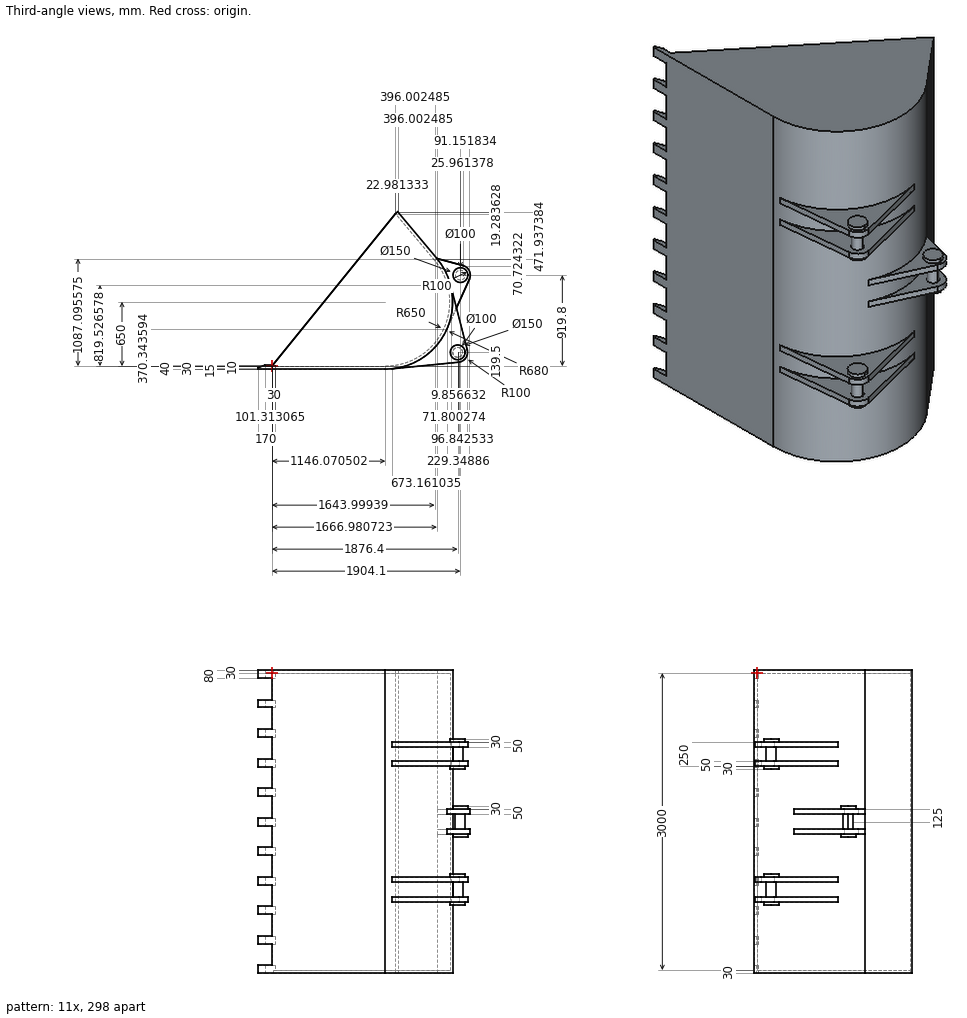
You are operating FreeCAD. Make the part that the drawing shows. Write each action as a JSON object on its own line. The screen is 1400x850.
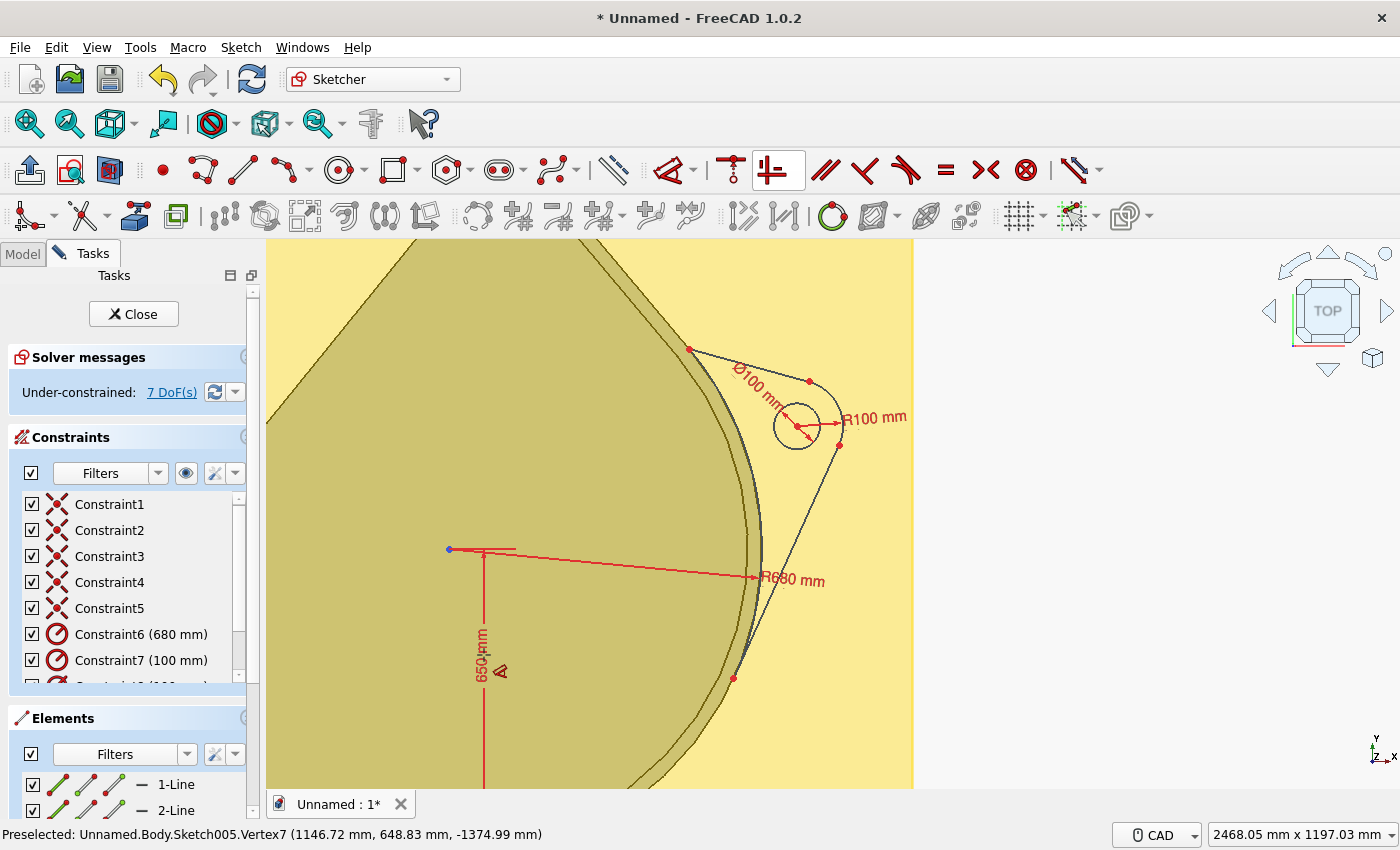
{"action": "left_click", "coordinate": [797, 426]}
{"action": "left_click", "coordinate": [831, 517]}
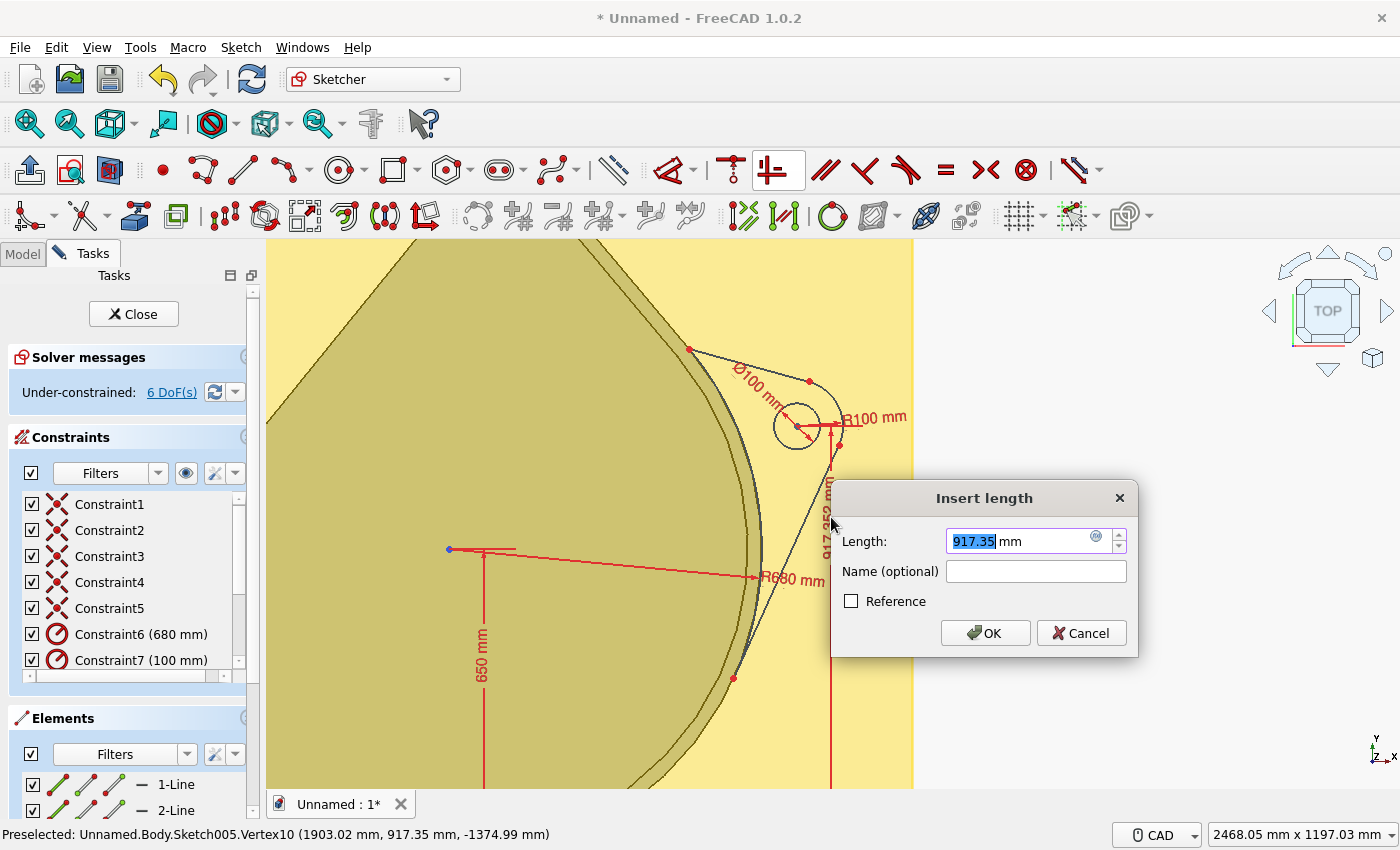
{"action": "type", "text": "919.8"}
{"action": "key", "text": "Return"}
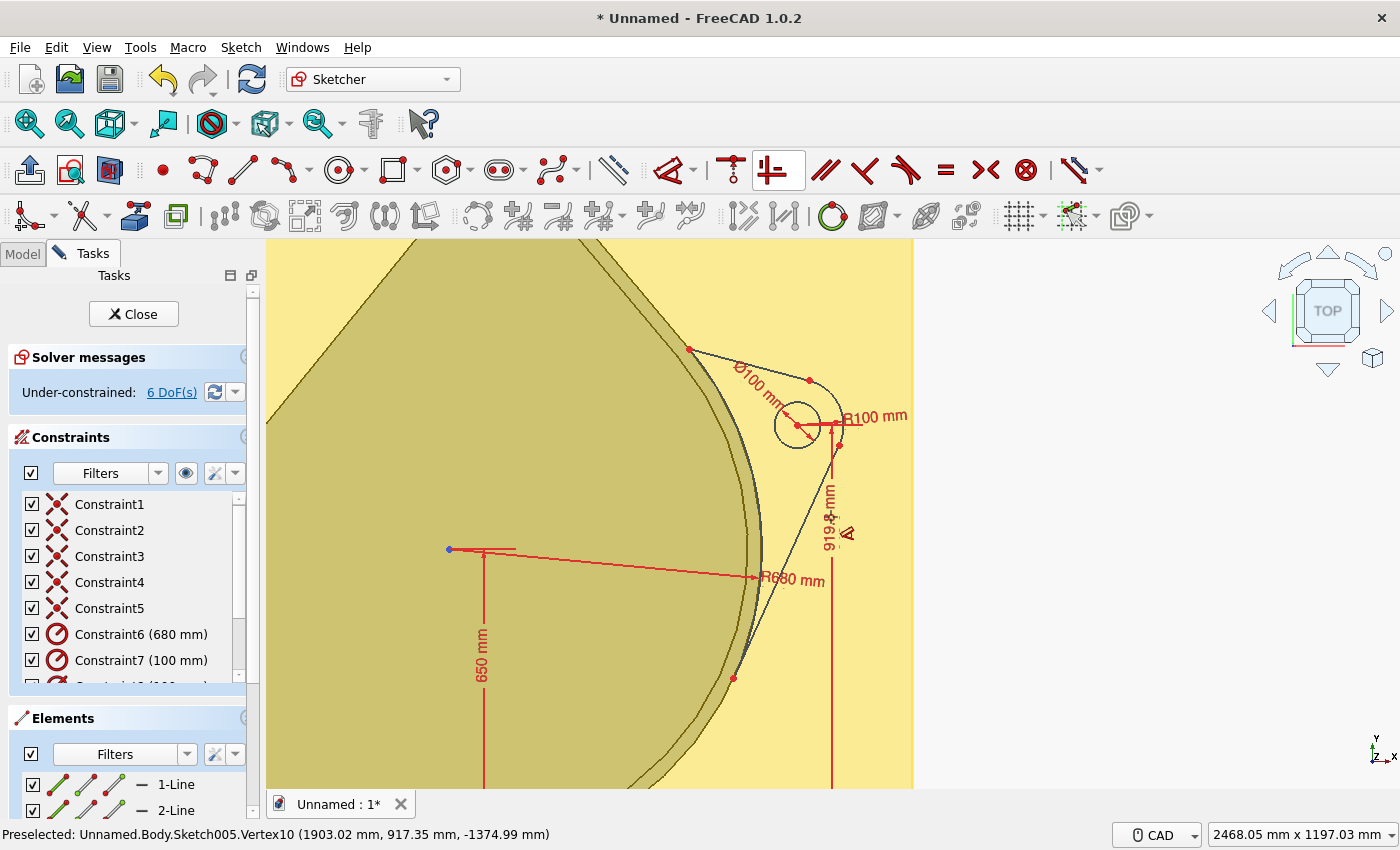
{"action": "left_click", "coordinate": [798, 425]}
{"action": "left_click", "coordinate": [546, 391]}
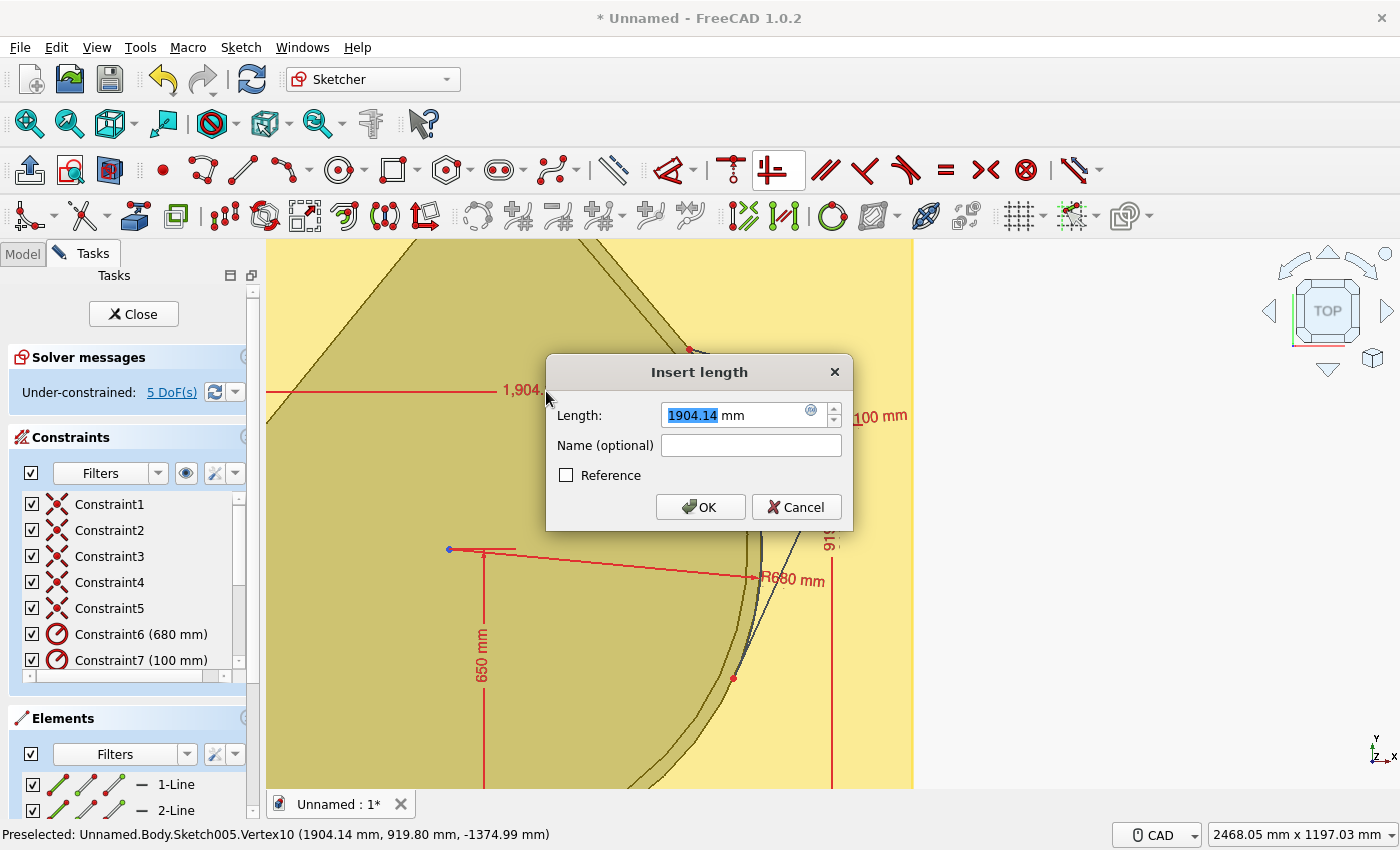
{"action": "type", "text": "1904.1"}
{"action": "key", "text": "Return"}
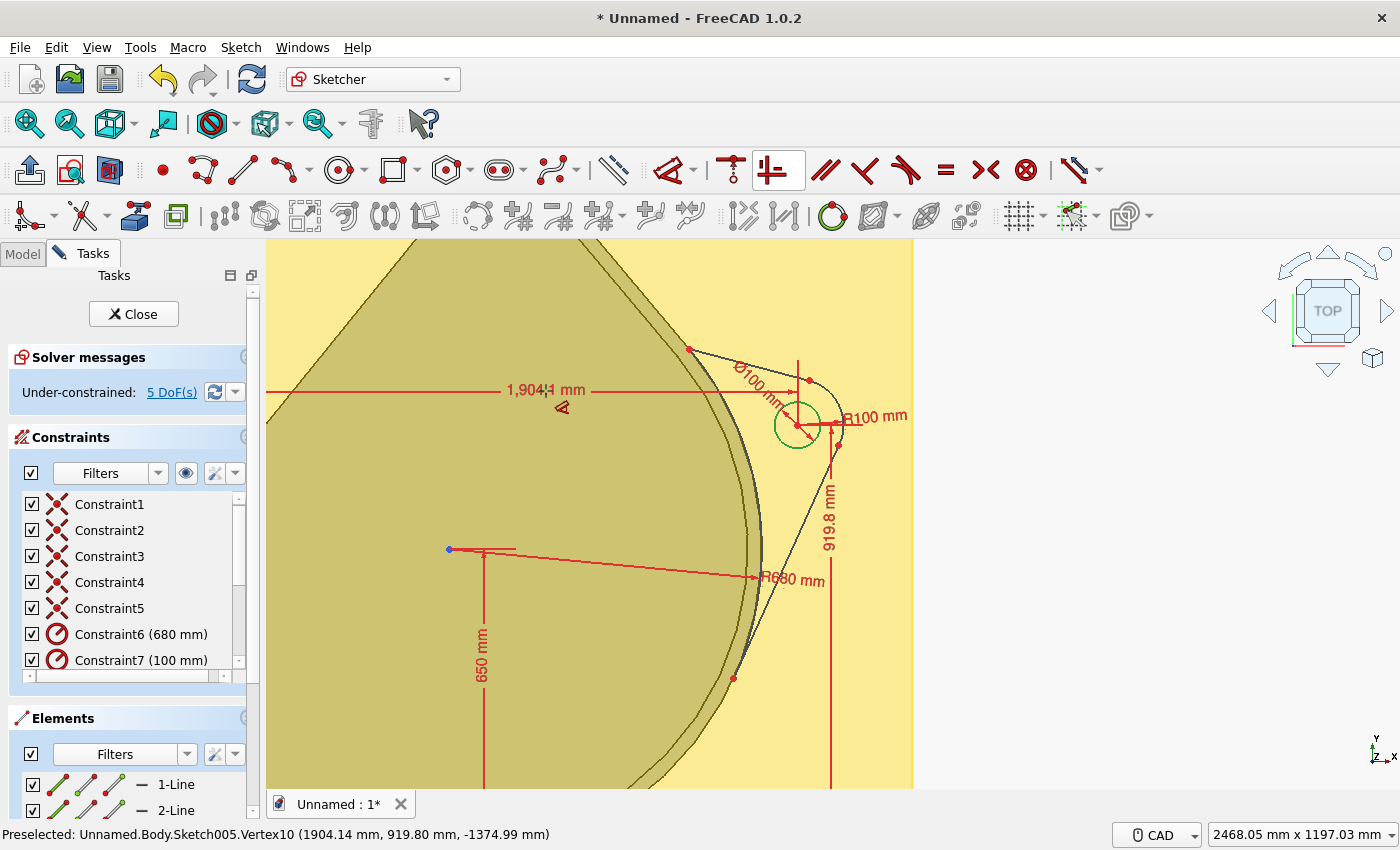
{"action": "scroll", "coordinate": [773, 371], "scroll_direction": "up", "scroll_amount": 2}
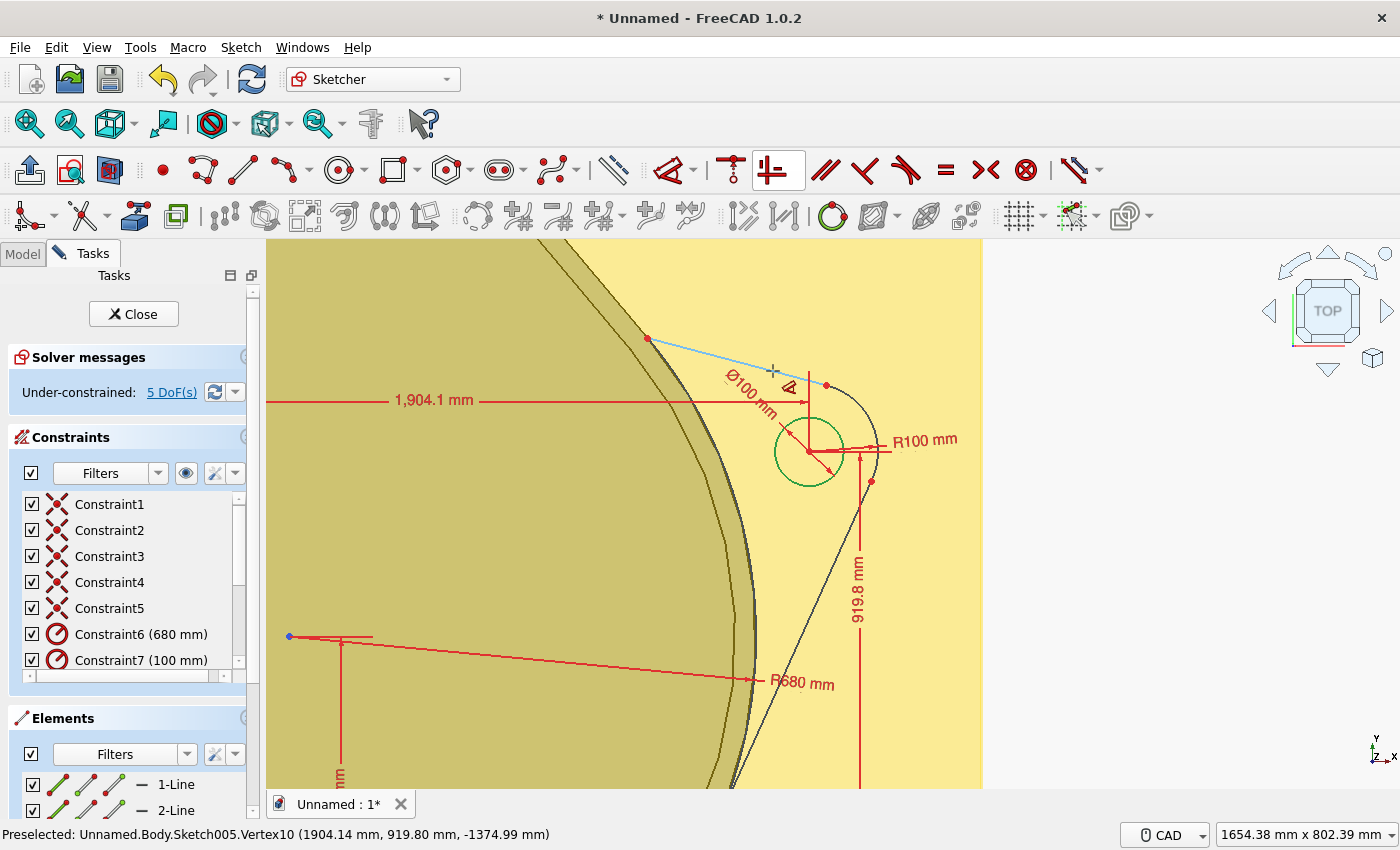
{"action": "left_click", "coordinate": [773, 371]}
{"action": "left_click", "coordinate": [614, 362]}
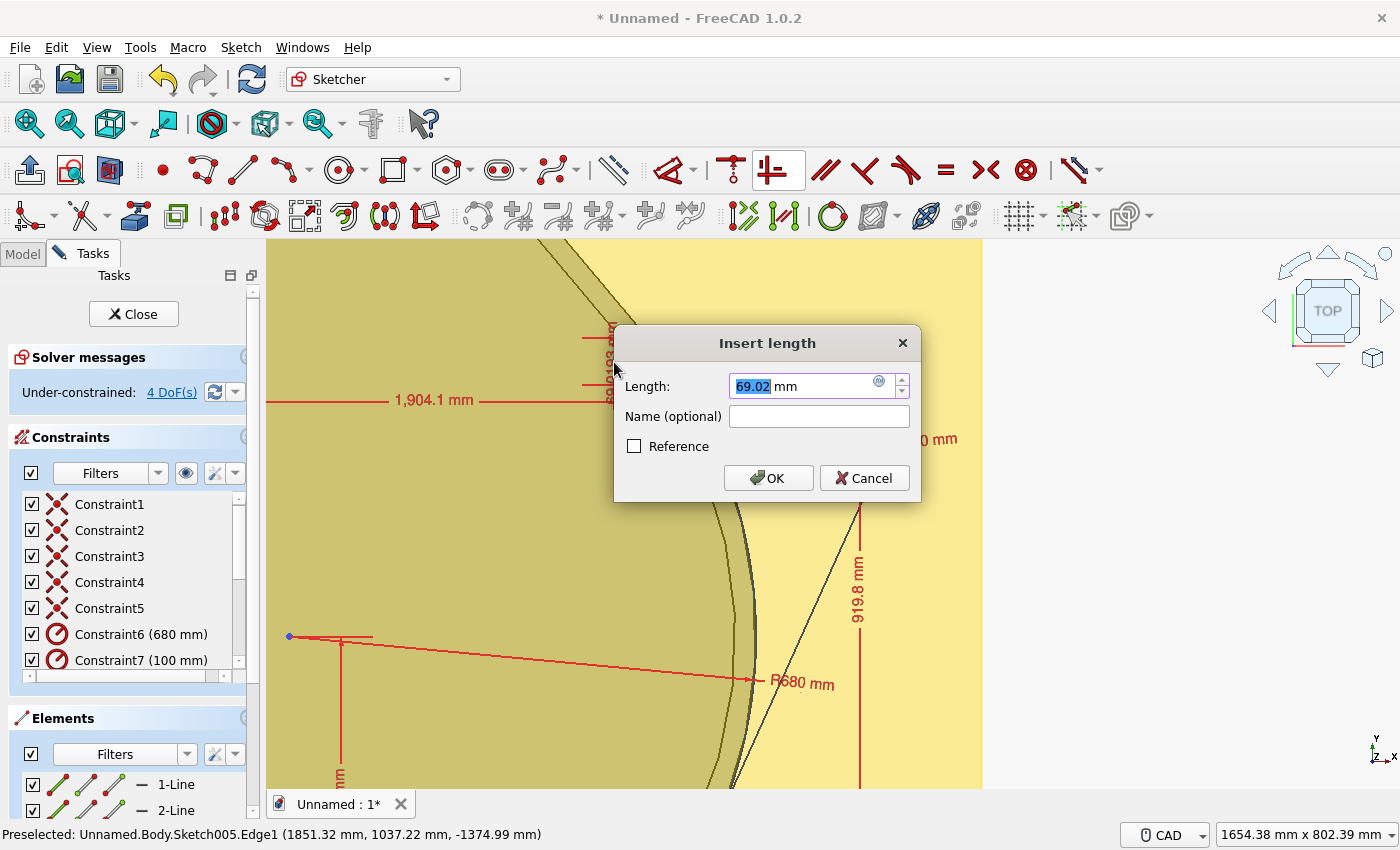
{"action": "type", "text": "70.724322"}
{"action": "key", "text": "Return"}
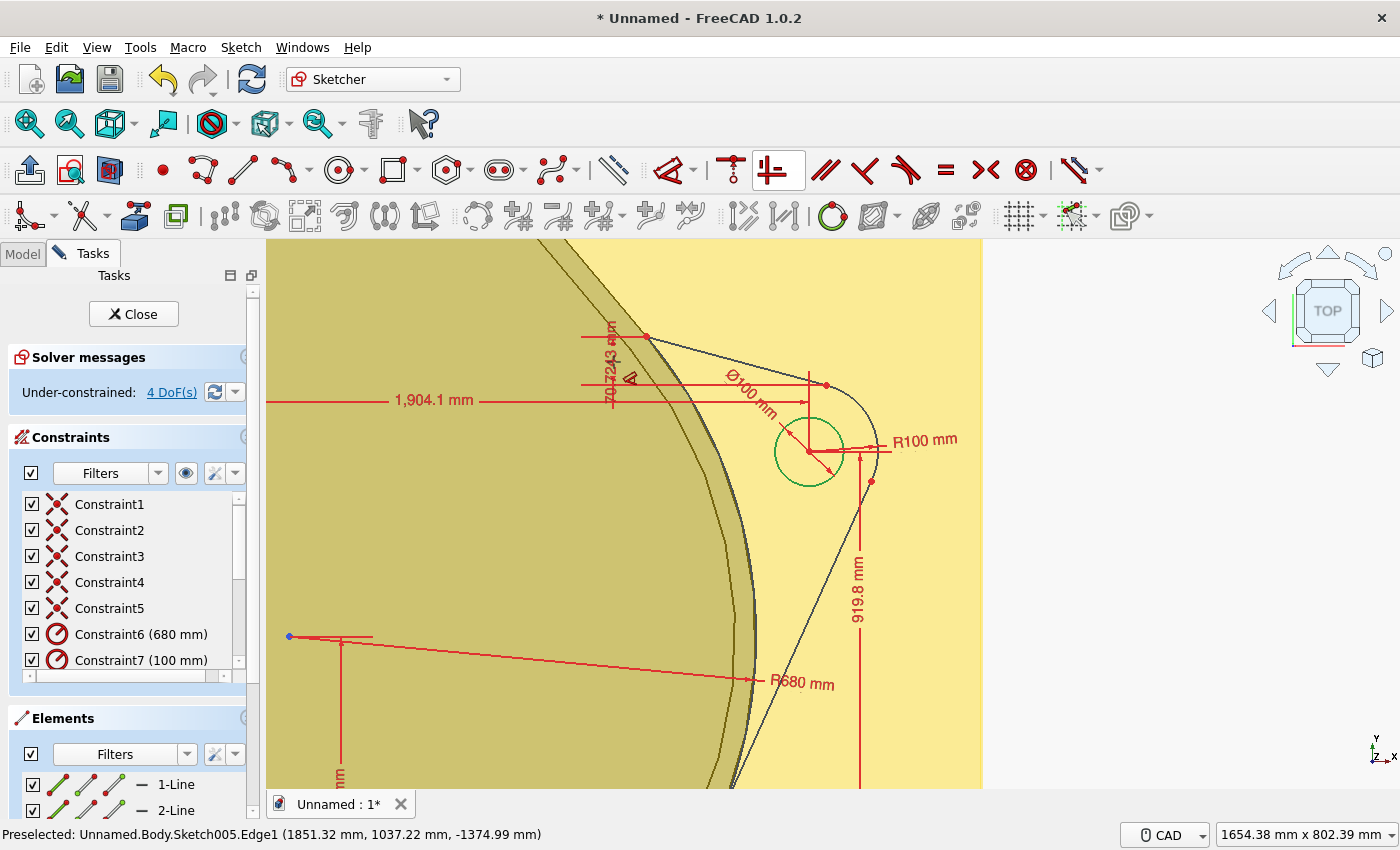
{"action": "left_click", "coordinate": [761, 726]}
{"action": "left_click", "coordinate": [793, 447]}